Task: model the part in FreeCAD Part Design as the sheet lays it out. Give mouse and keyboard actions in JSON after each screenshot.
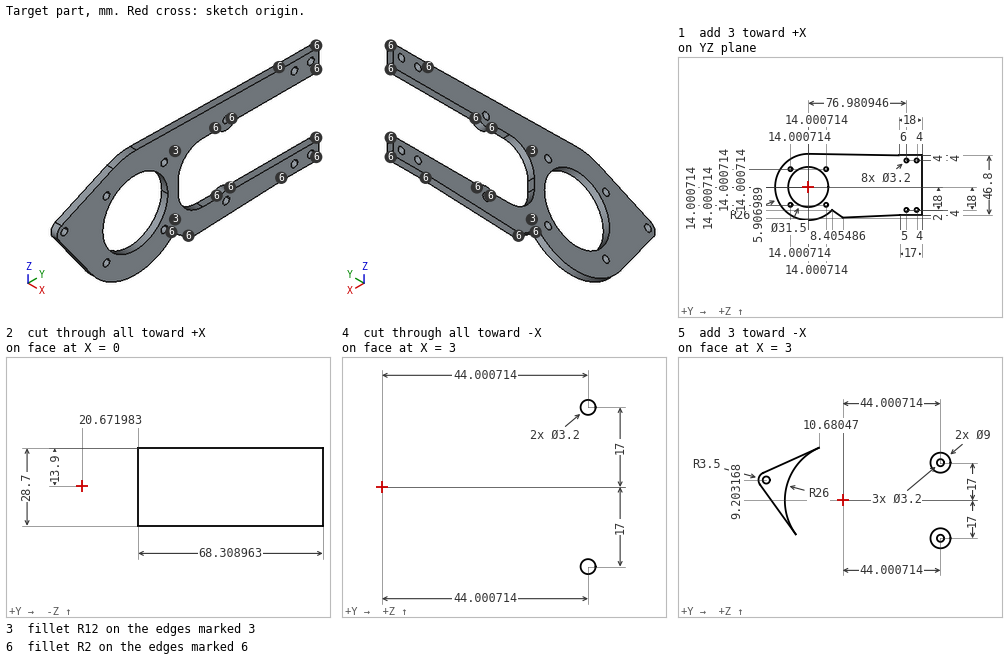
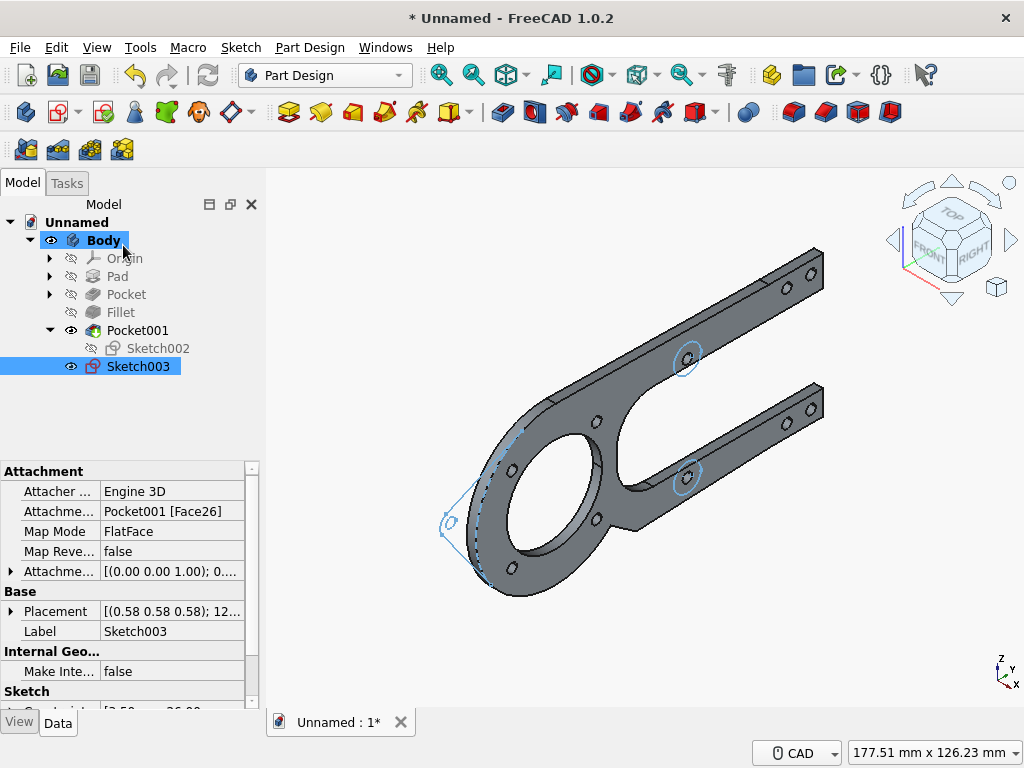
{"action": "left_click", "coordinate": [290, 112]}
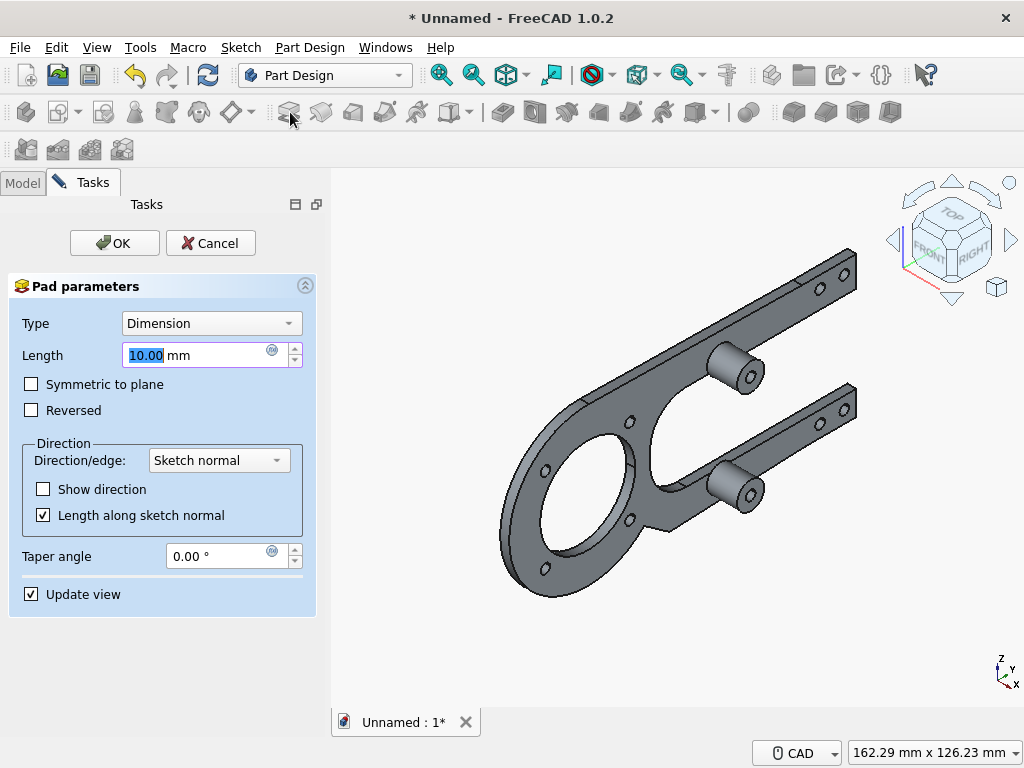
{"action": "type", "text": "3"}
{"action": "key", "text": "Tab"}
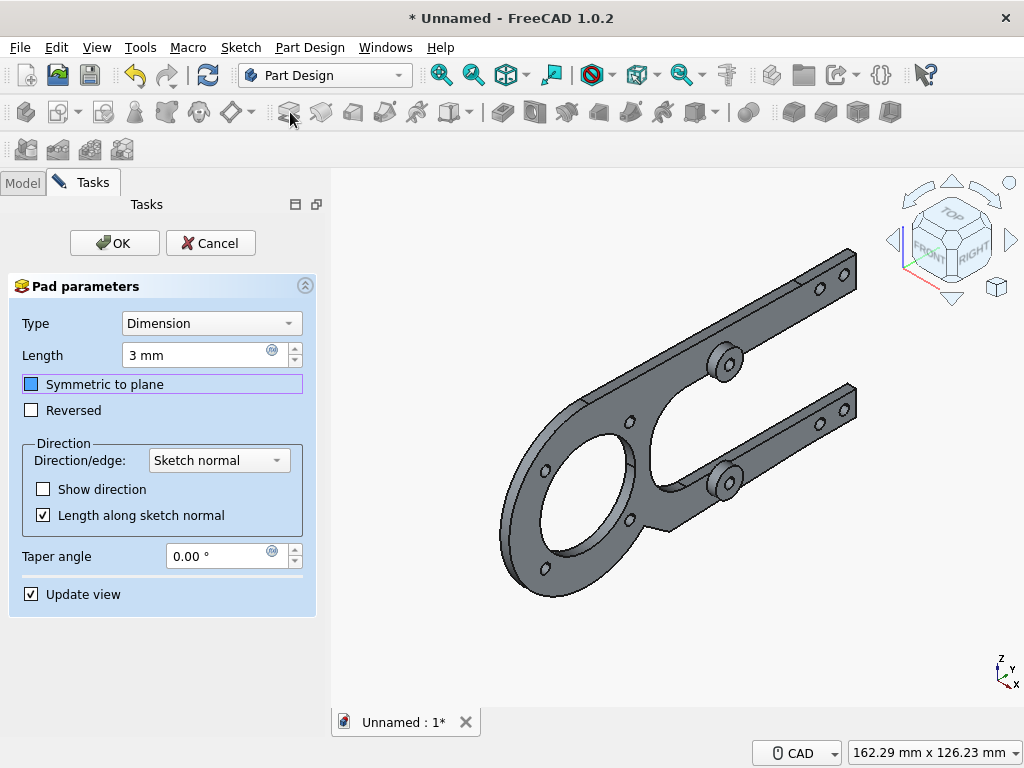
{"action": "left_click", "coordinate": [30, 410]}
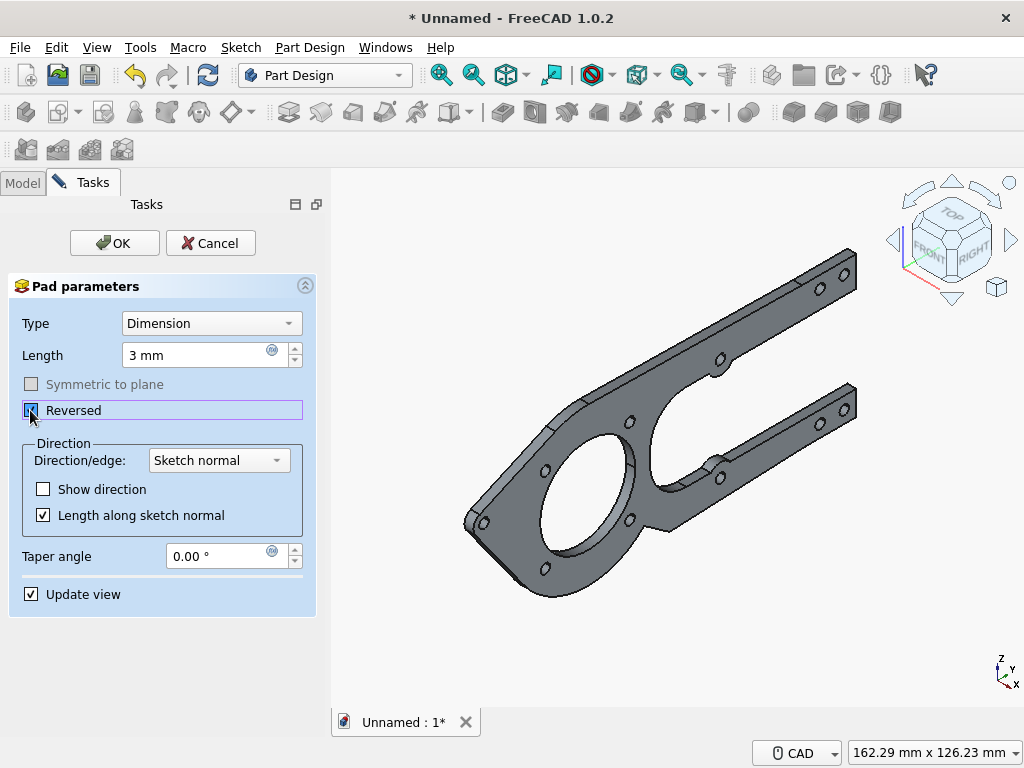
{"action": "left_click", "coordinate": [115, 243]}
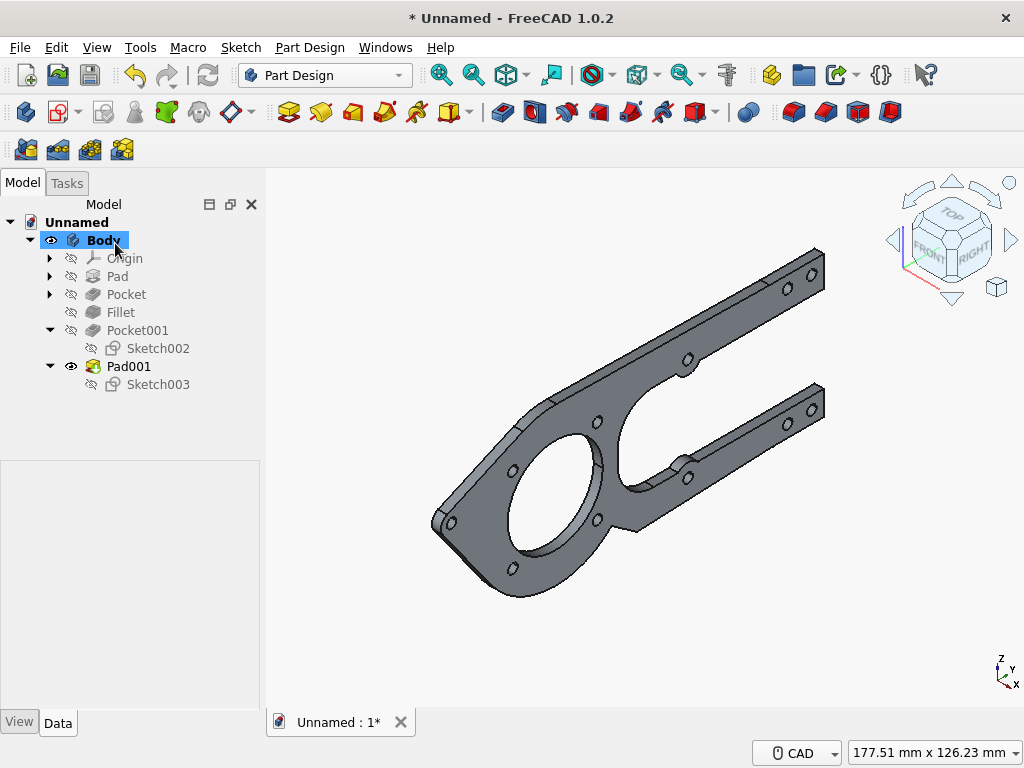
{"action": "scroll", "coordinate": [695, 357], "scroll_direction": "up", "scroll_amount": 6}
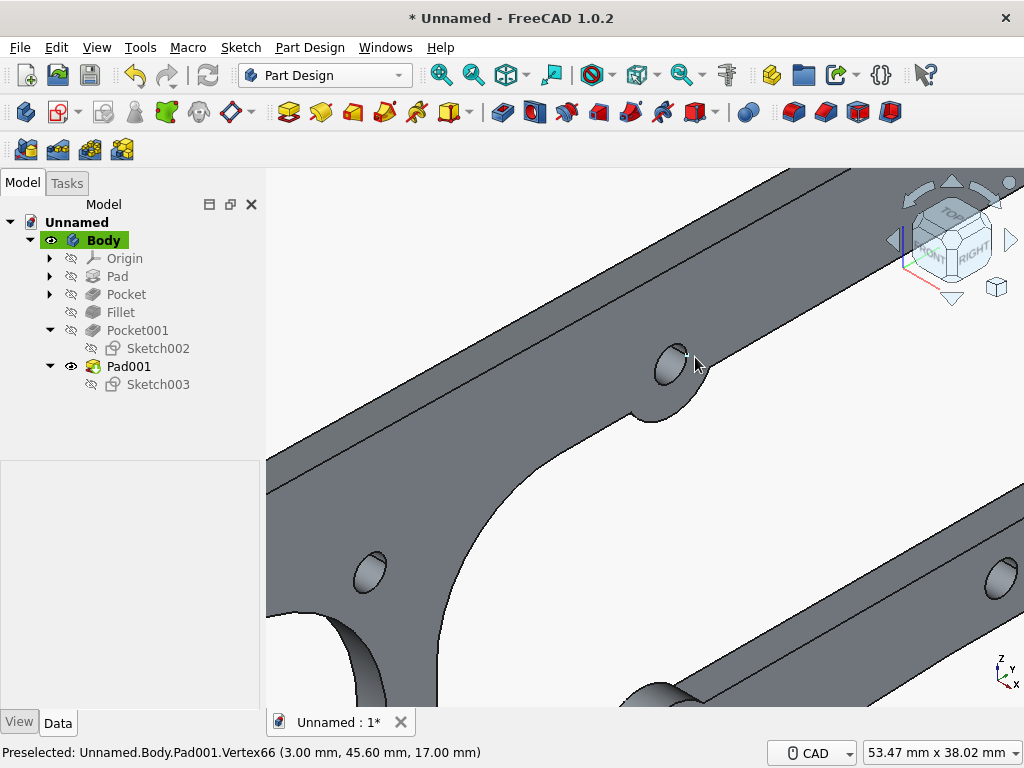
{"action": "left_click", "coordinate": [442, 76]}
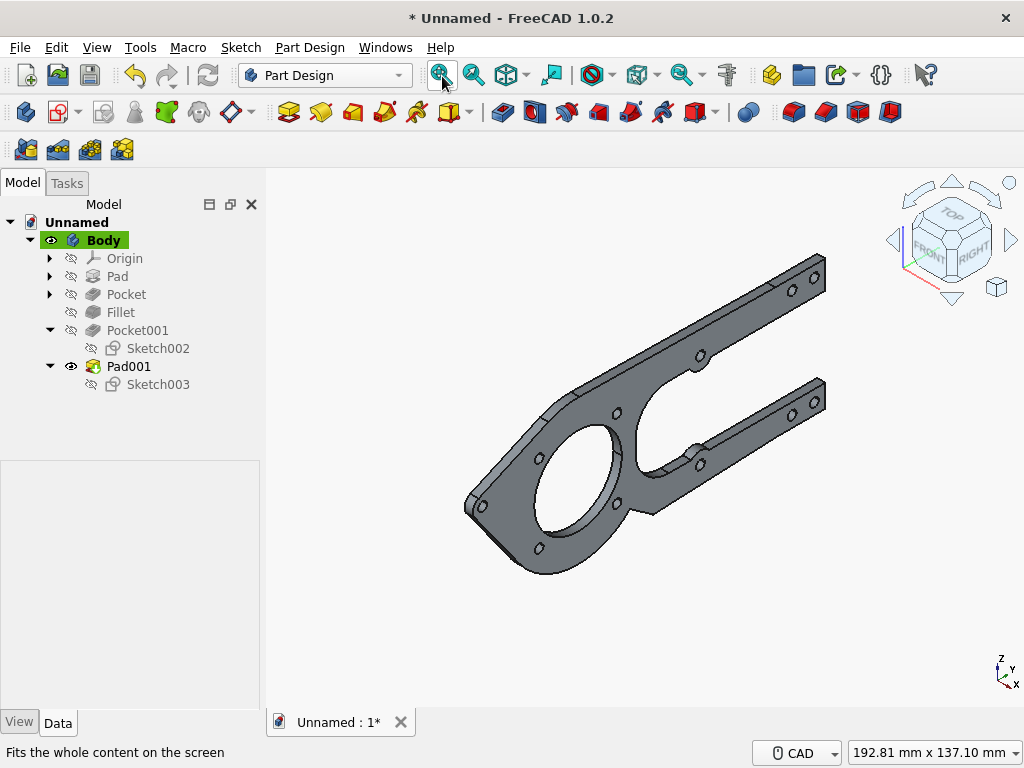
{"action": "key", "text": "2"}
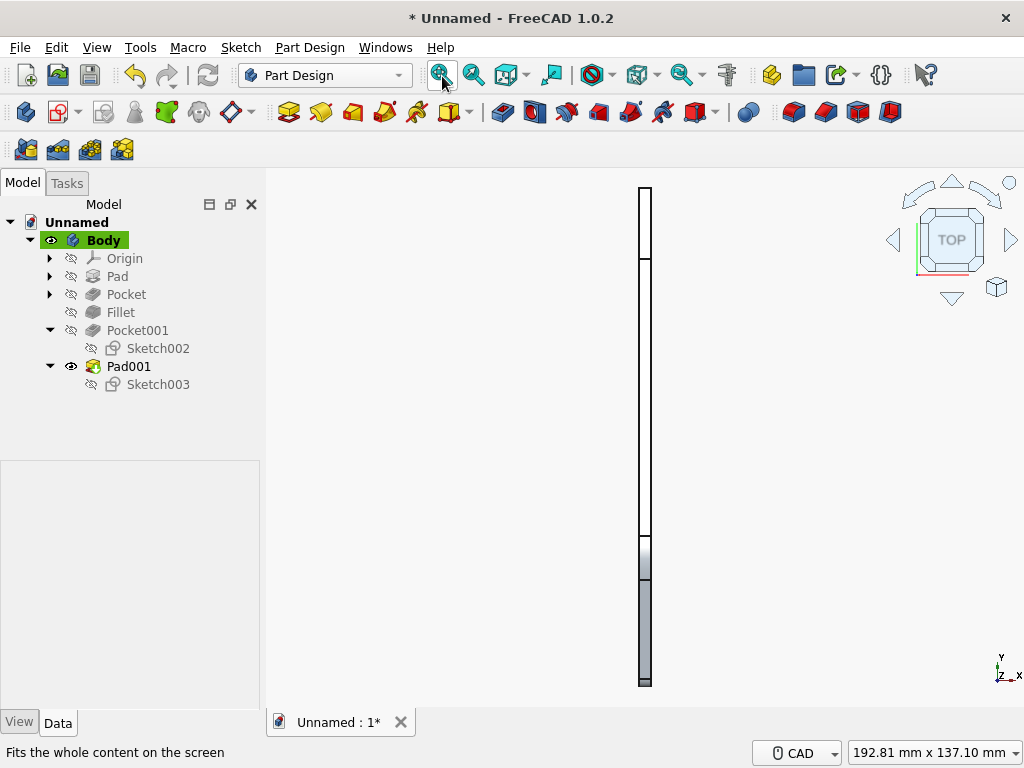
{"action": "scroll", "coordinate": [645, 349], "scroll_direction": "up", "scroll_amount": 7}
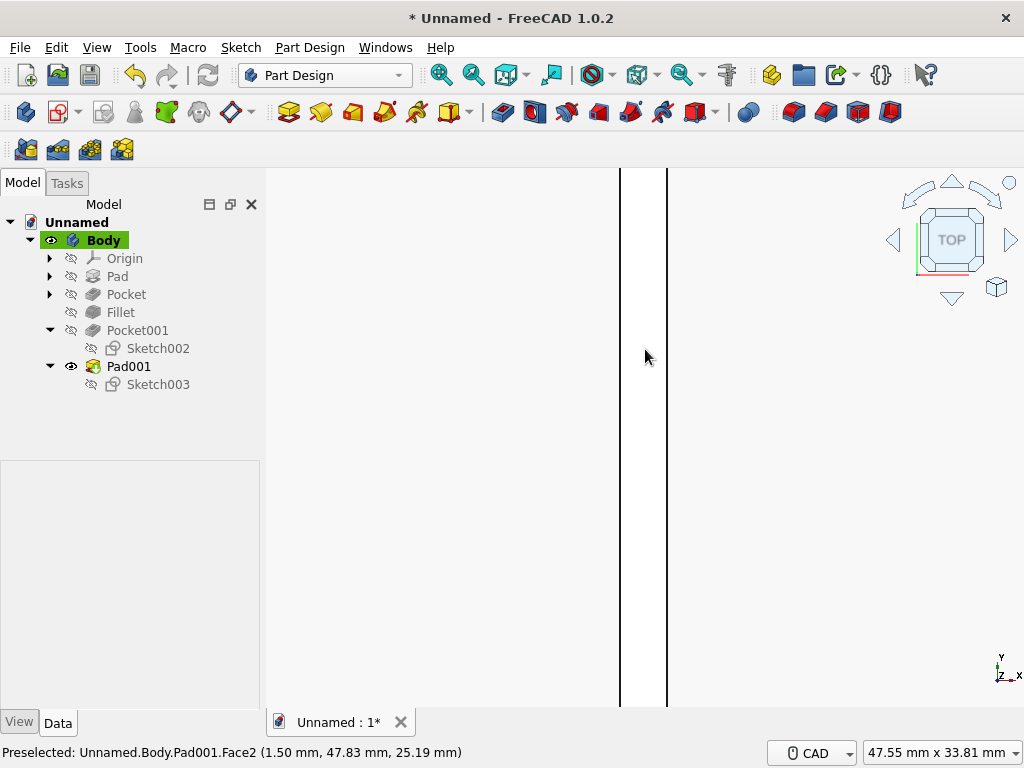
{"action": "left_click", "coordinate": [442, 76]}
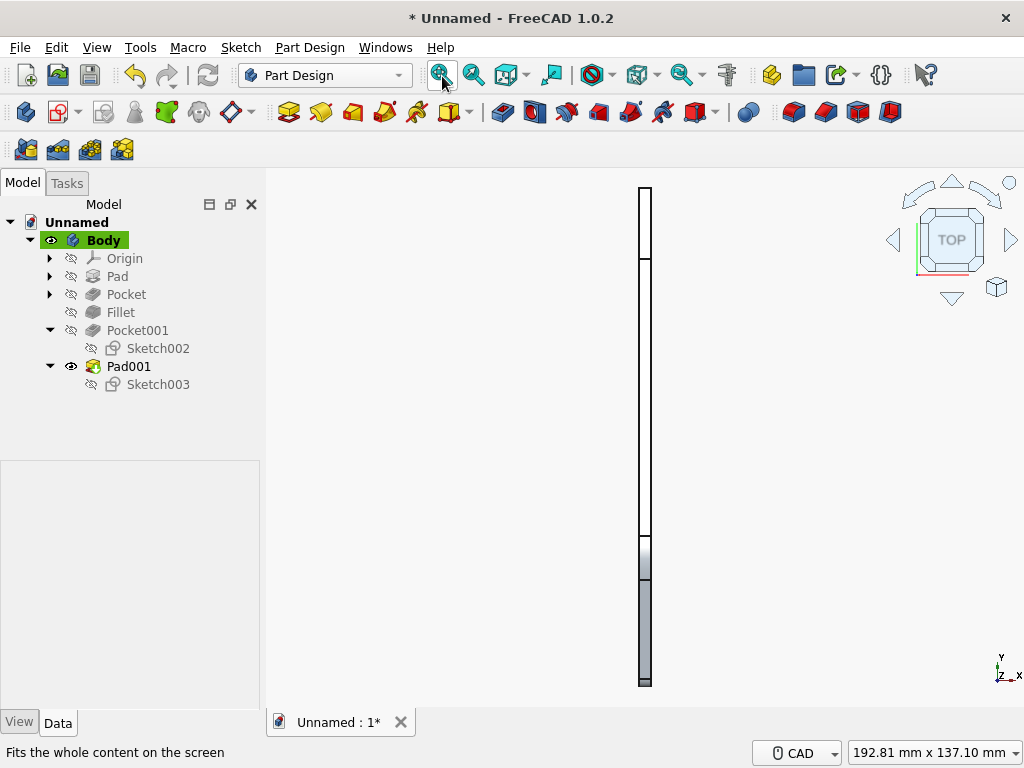
{"action": "key", "text": "0"}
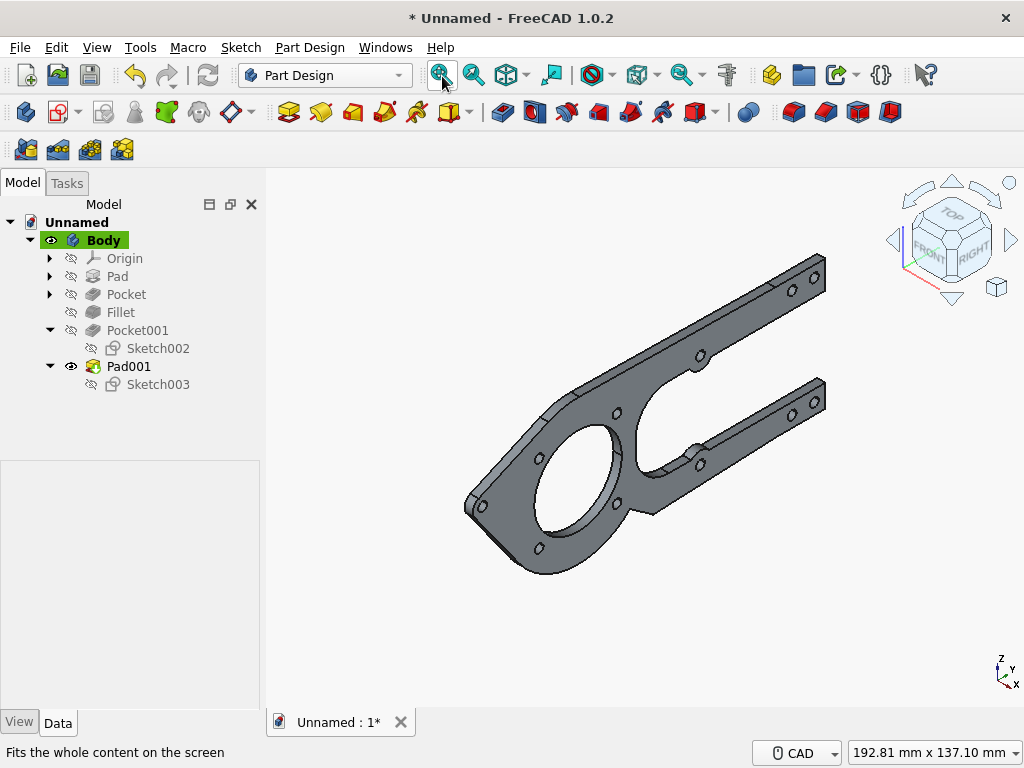
{"action": "scroll", "coordinate": [707, 353], "scroll_direction": "up", "scroll_amount": 7}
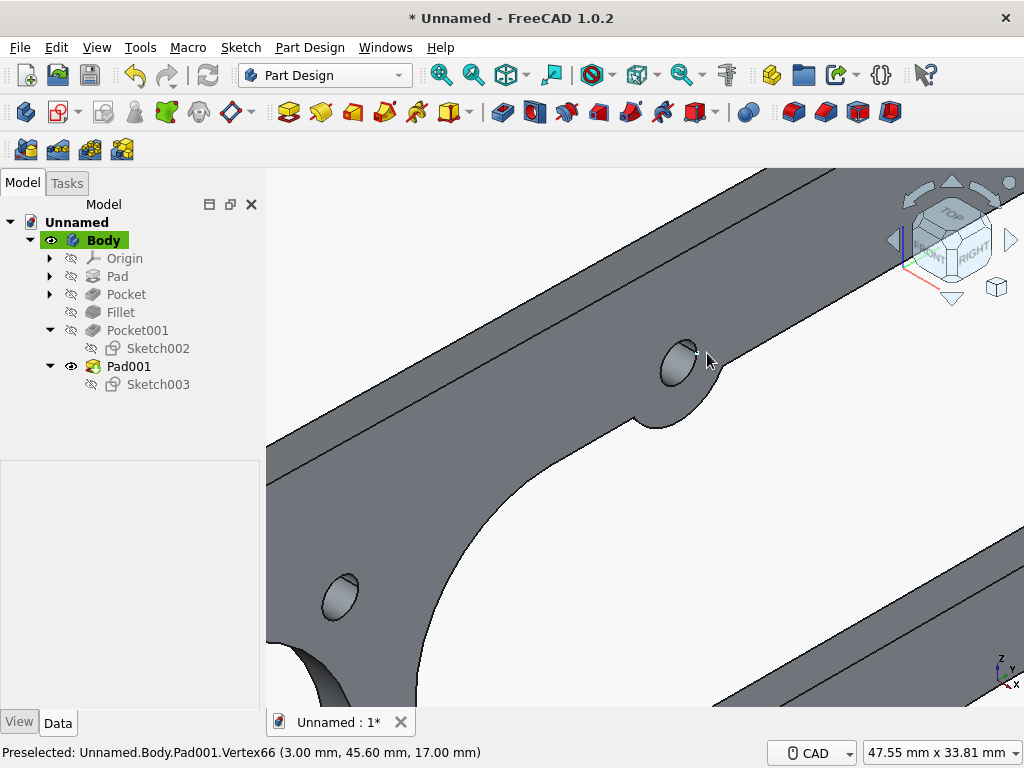
{"action": "left_click", "coordinate": [442, 76]}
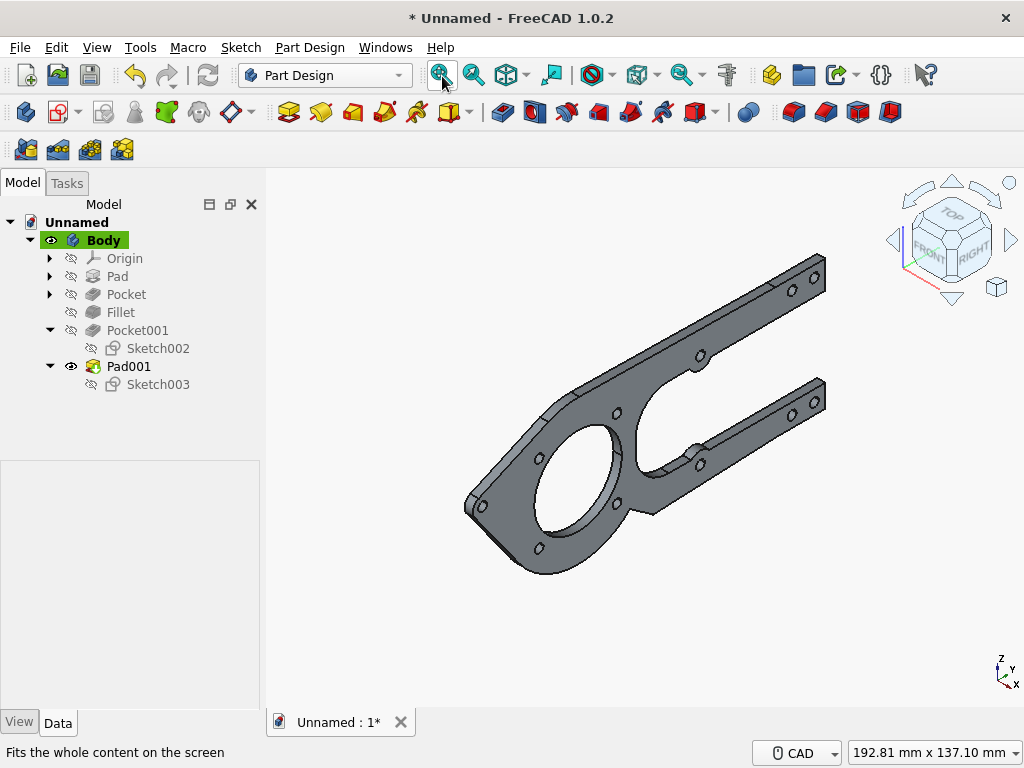
{"action": "key", "text": "1"}